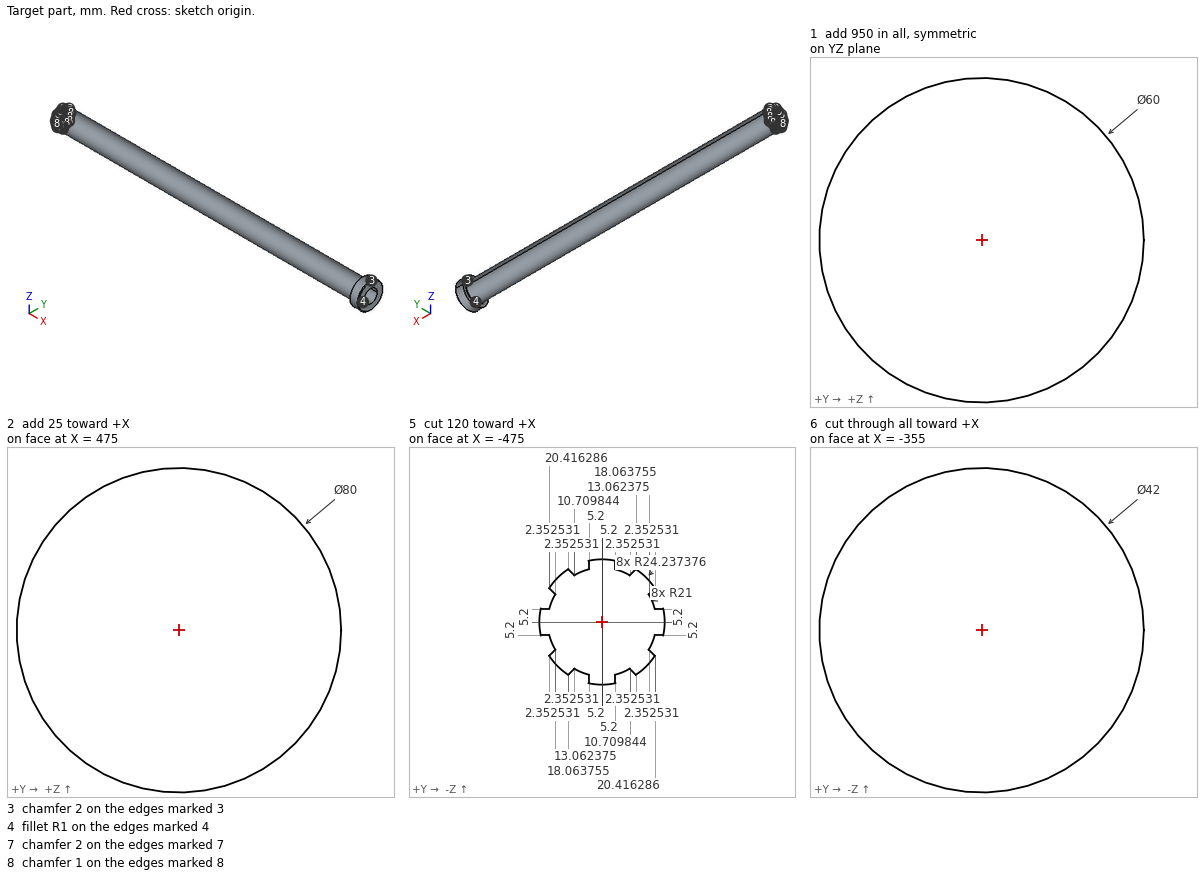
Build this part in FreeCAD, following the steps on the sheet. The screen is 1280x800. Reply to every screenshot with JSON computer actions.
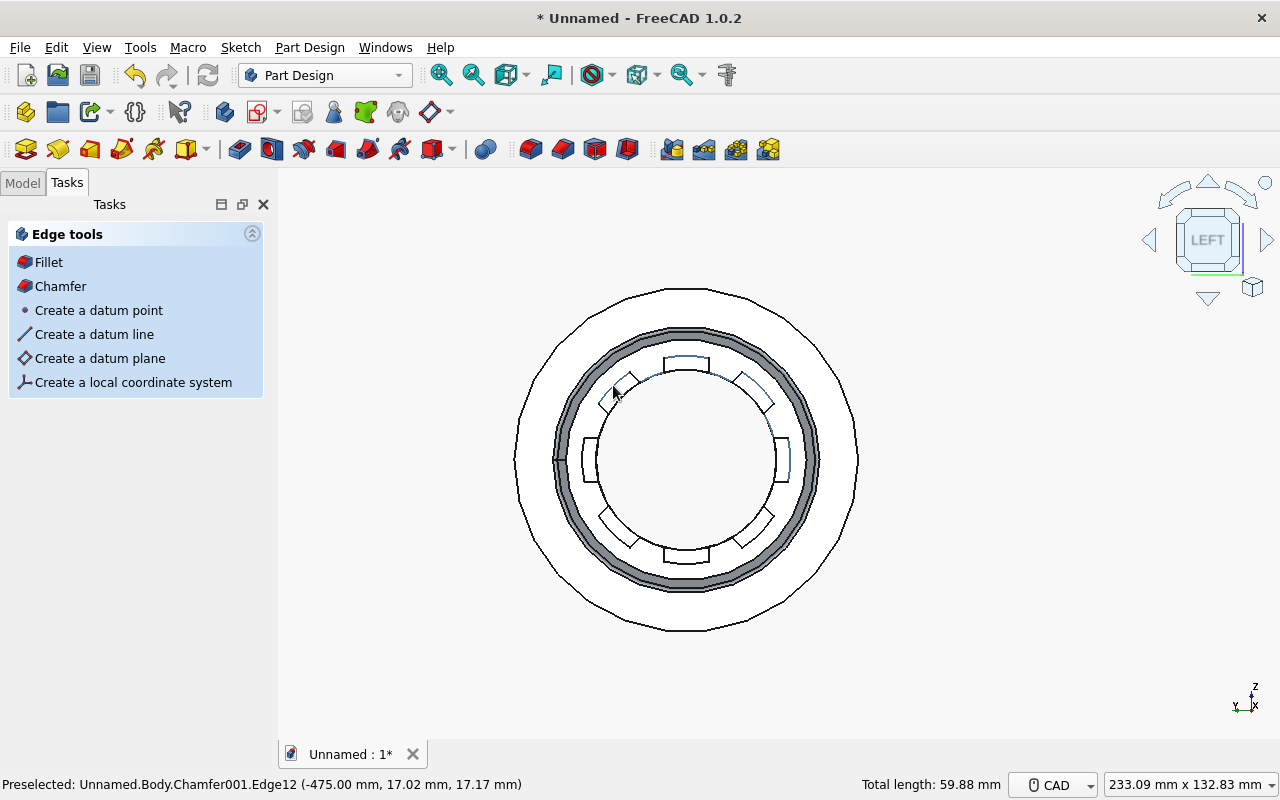
{"action": "left_click", "coordinate": [603, 424], "text": "ctrl"}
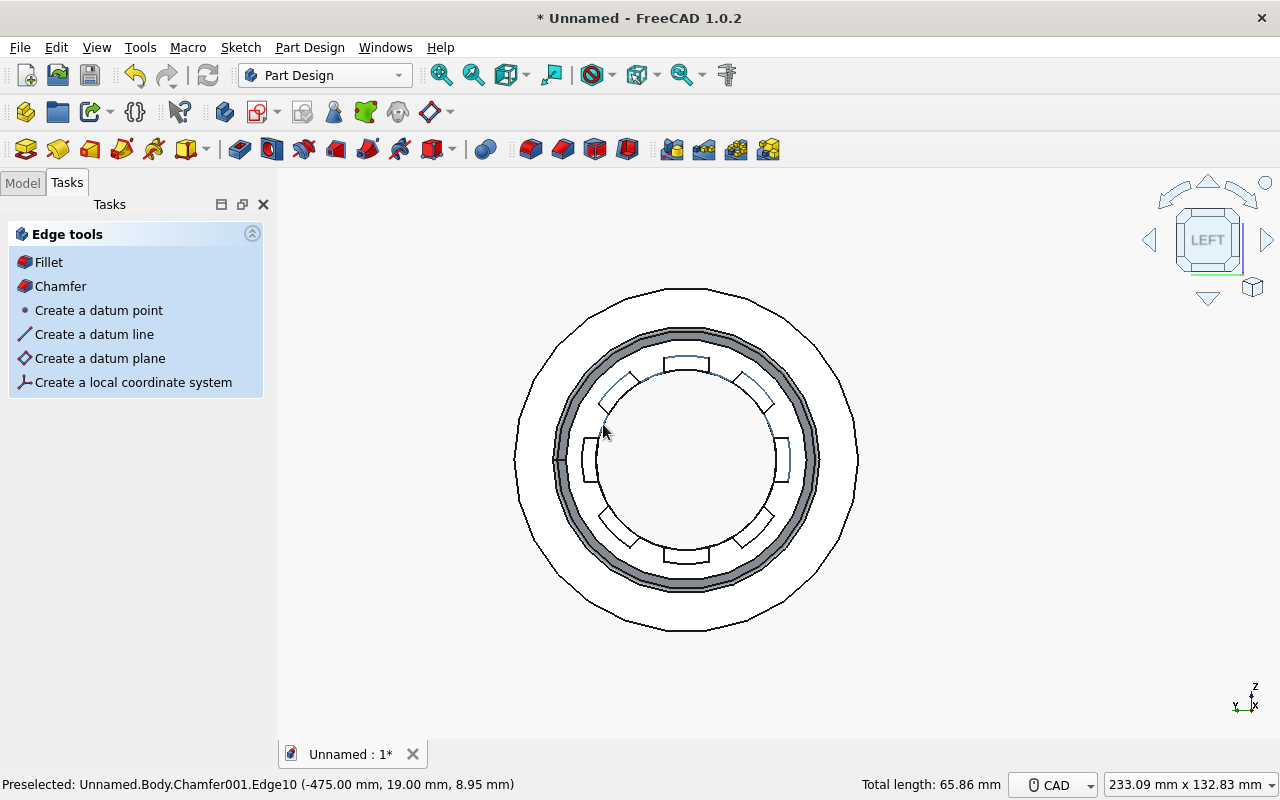
{"action": "left_click", "coordinate": [582, 459], "text": "ctrl"}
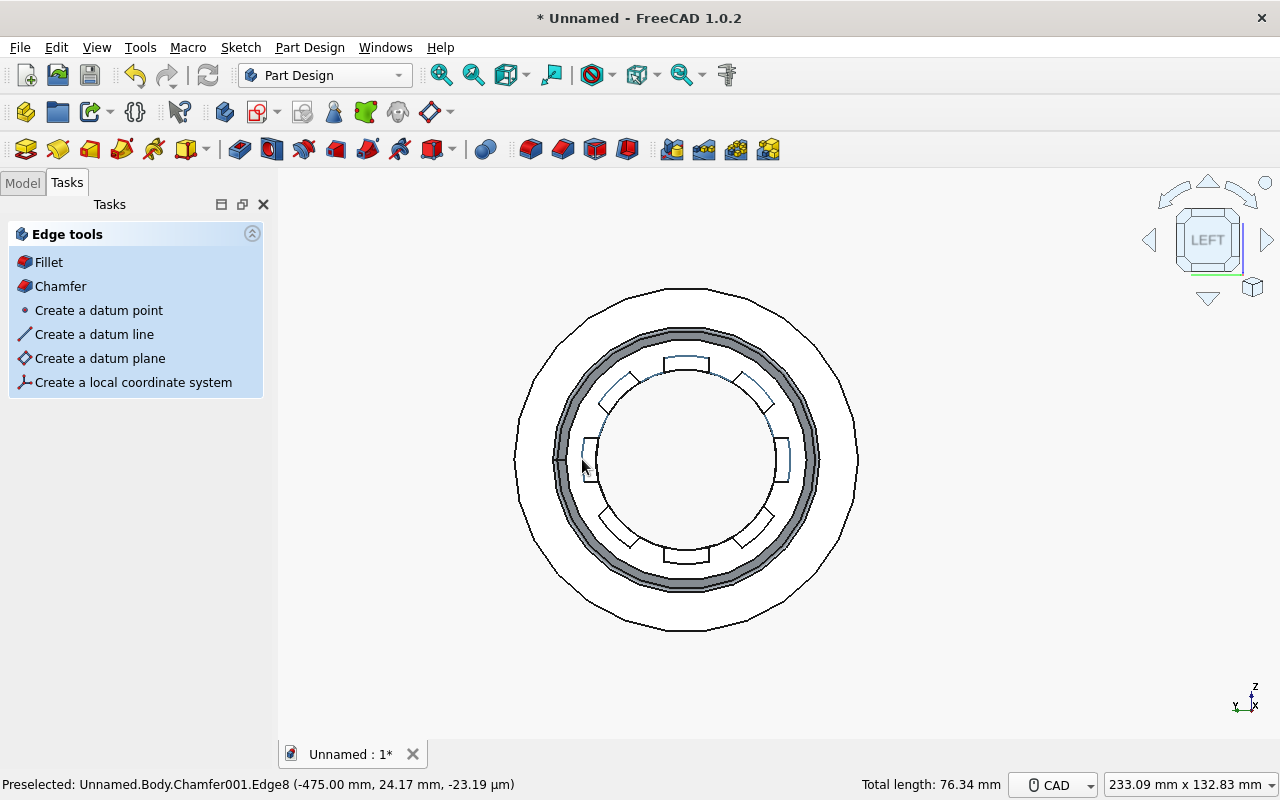
{"action": "left_click", "coordinate": [603, 493], "text": "ctrl"}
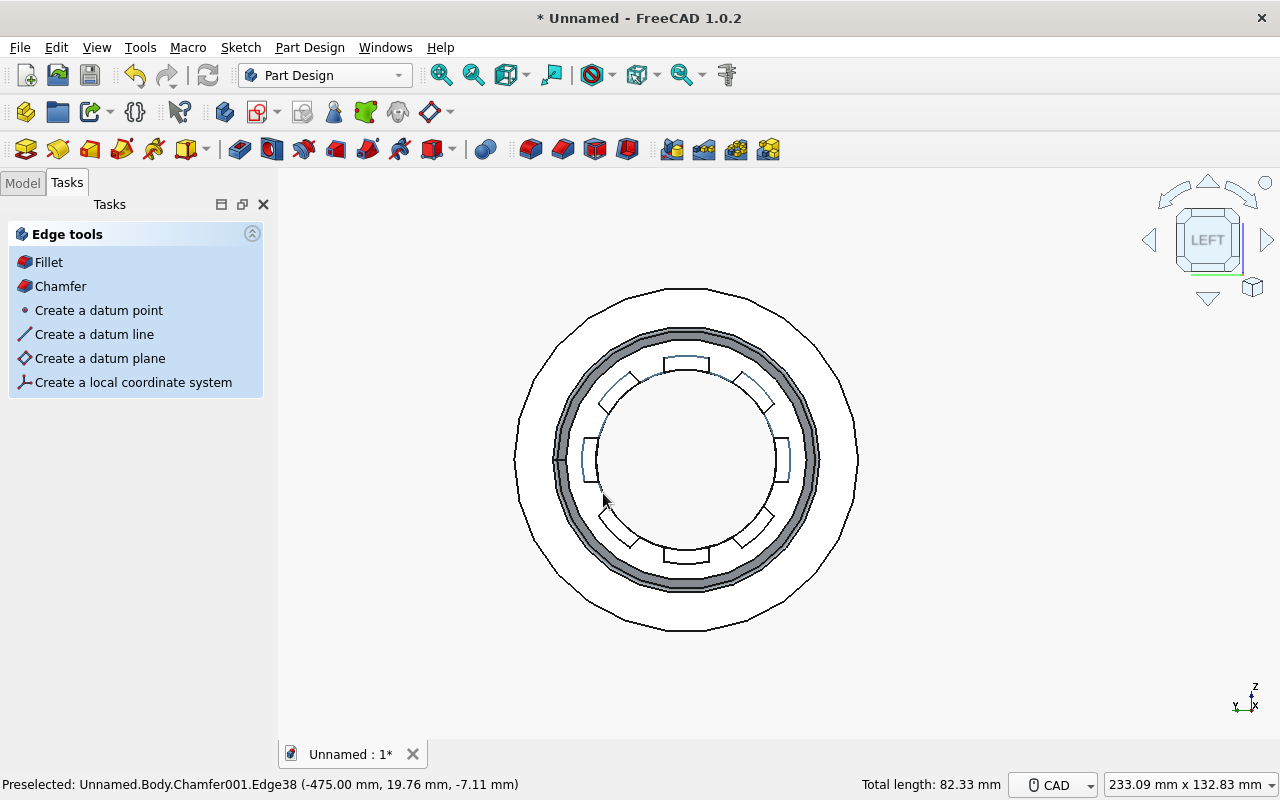
{"action": "left_click", "coordinate": [613, 533], "text": "ctrl"}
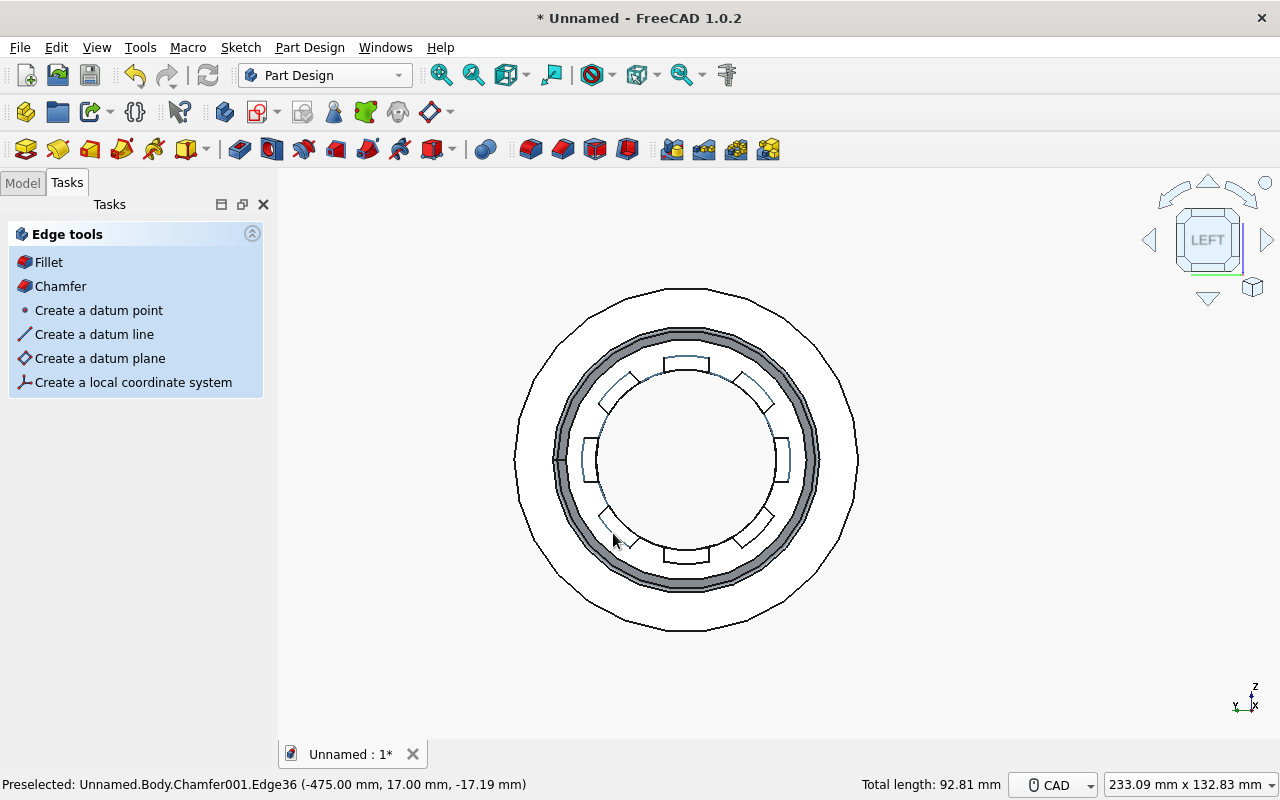
{"action": "left_click", "coordinate": [652, 542], "text": "ctrl"}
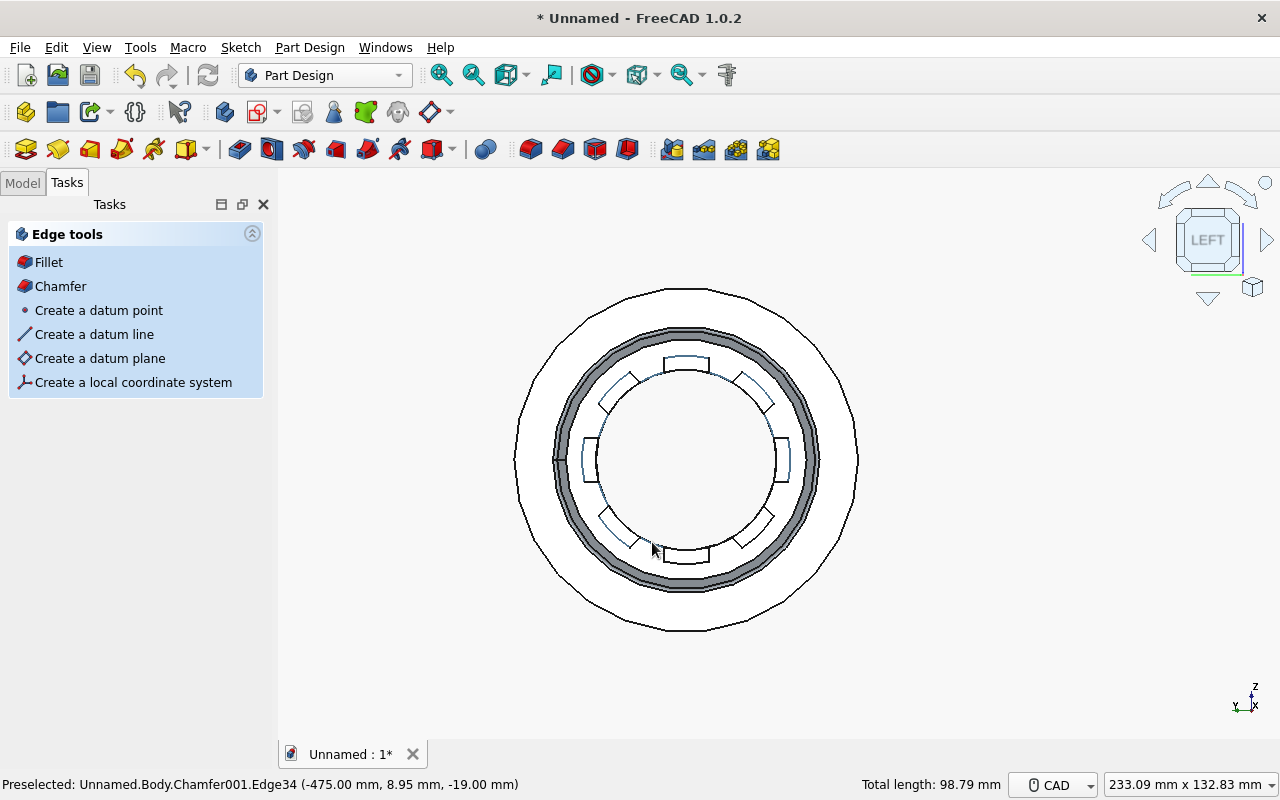
{"action": "left_click", "coordinate": [686, 563], "text": "ctrl"}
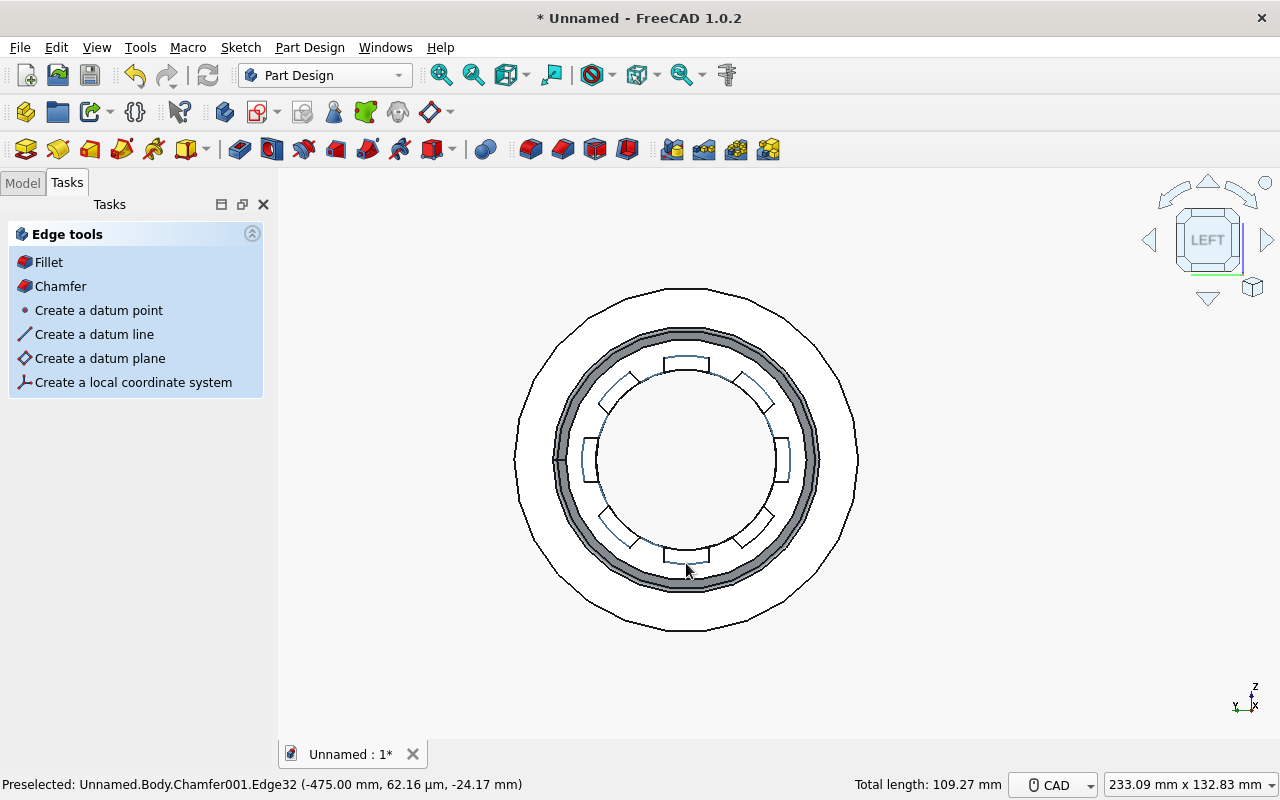
{"action": "left_click", "coordinate": [721, 542], "text": "ctrl"}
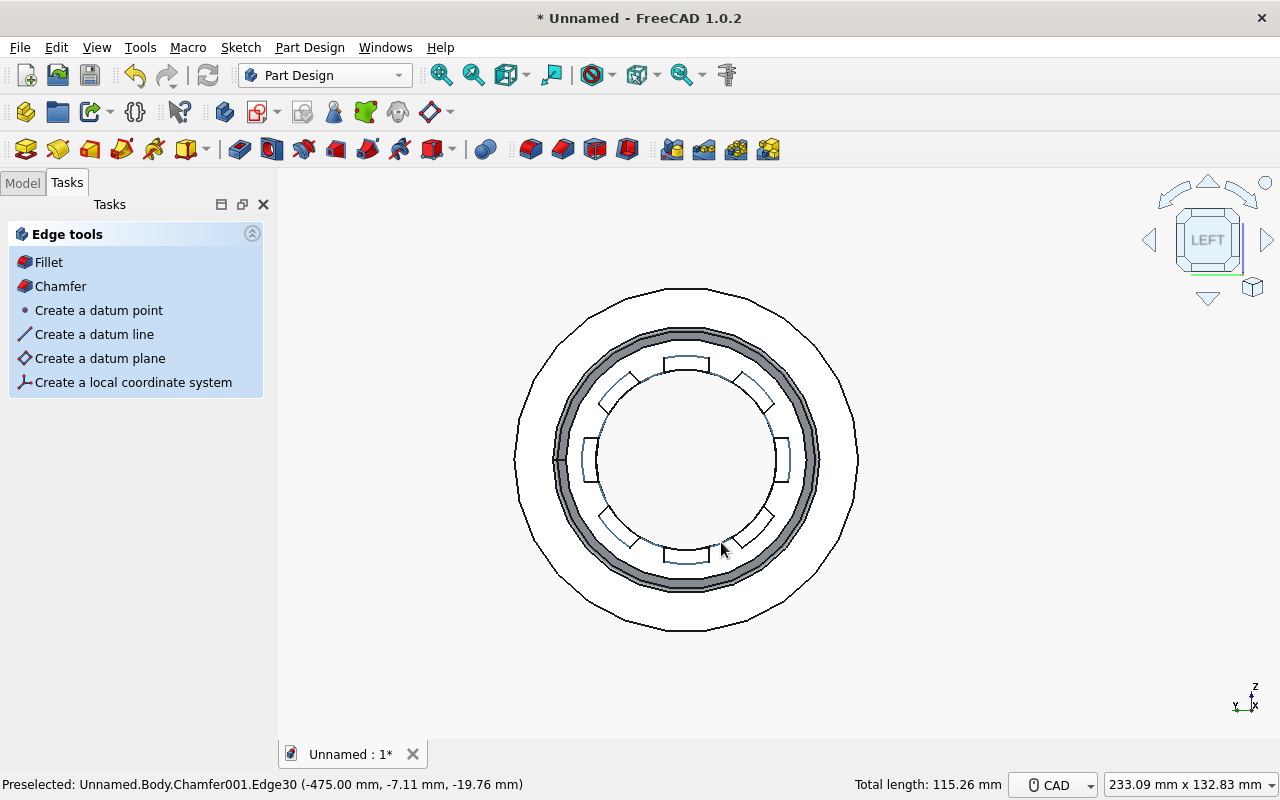
{"action": "left_click", "coordinate": [760, 533], "text": "ctrl"}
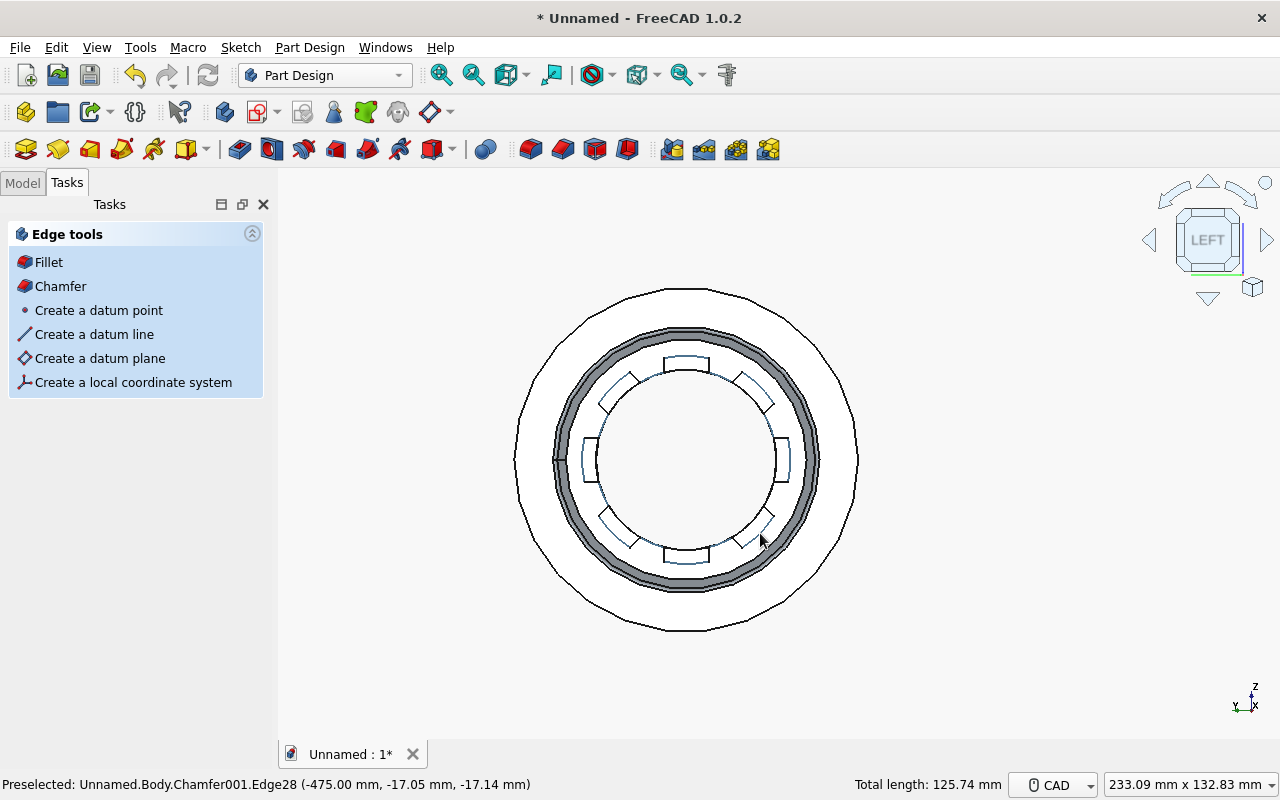
{"action": "left_click", "coordinate": [770, 493], "text": "ctrl"}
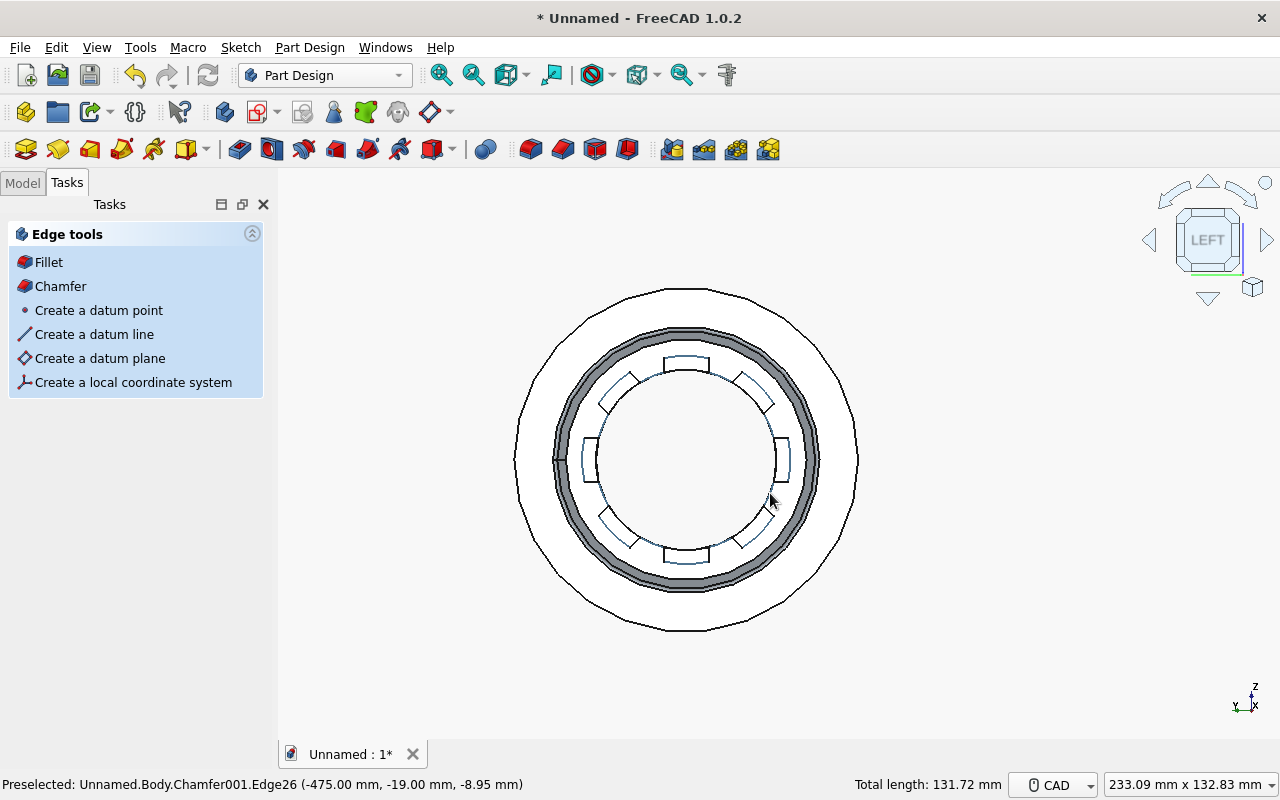
{"action": "left_click", "coordinate": [564, 150]}